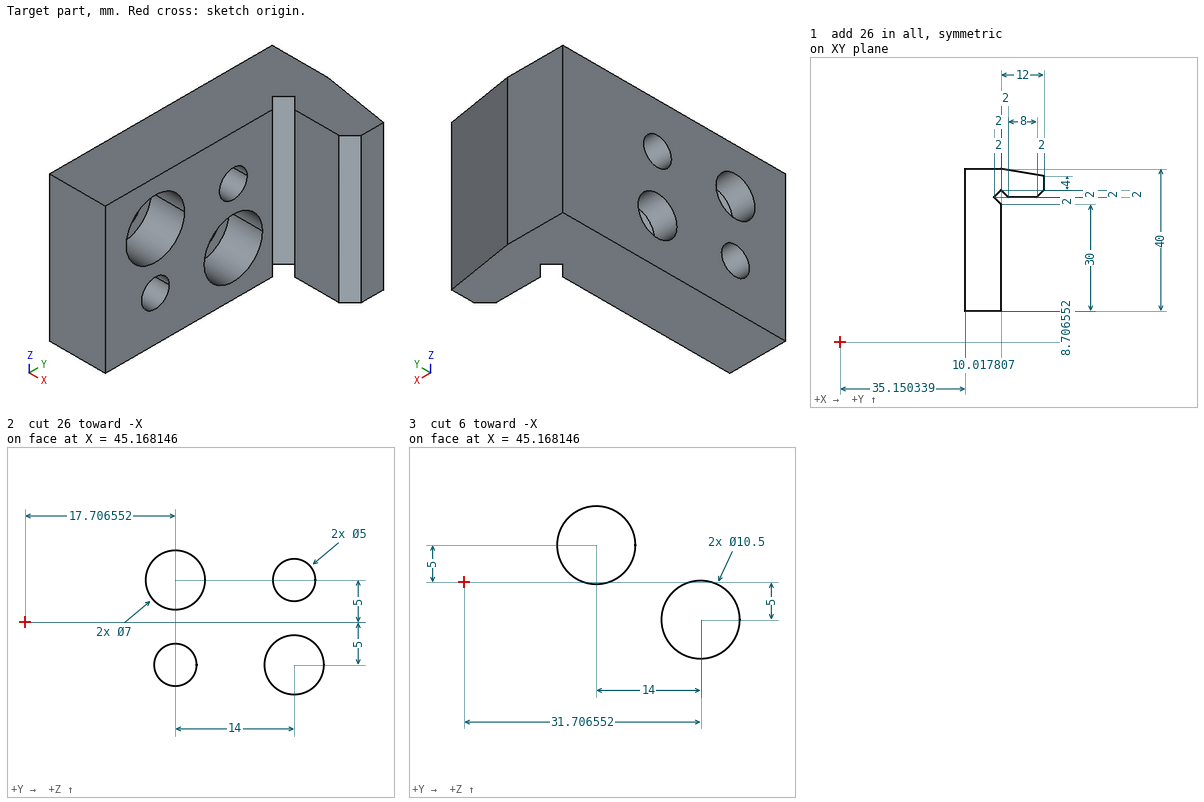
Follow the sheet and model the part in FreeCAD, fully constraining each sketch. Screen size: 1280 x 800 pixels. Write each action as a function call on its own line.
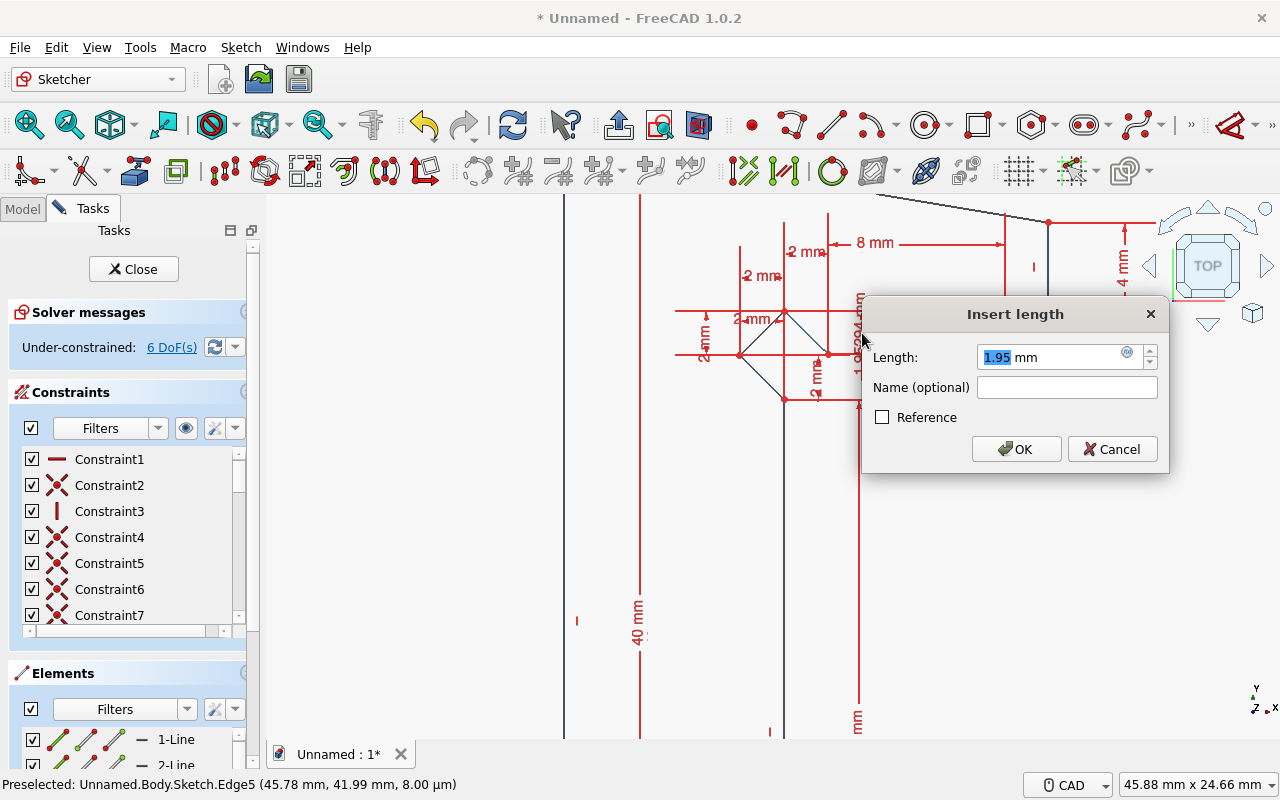
text(2)
key(Return)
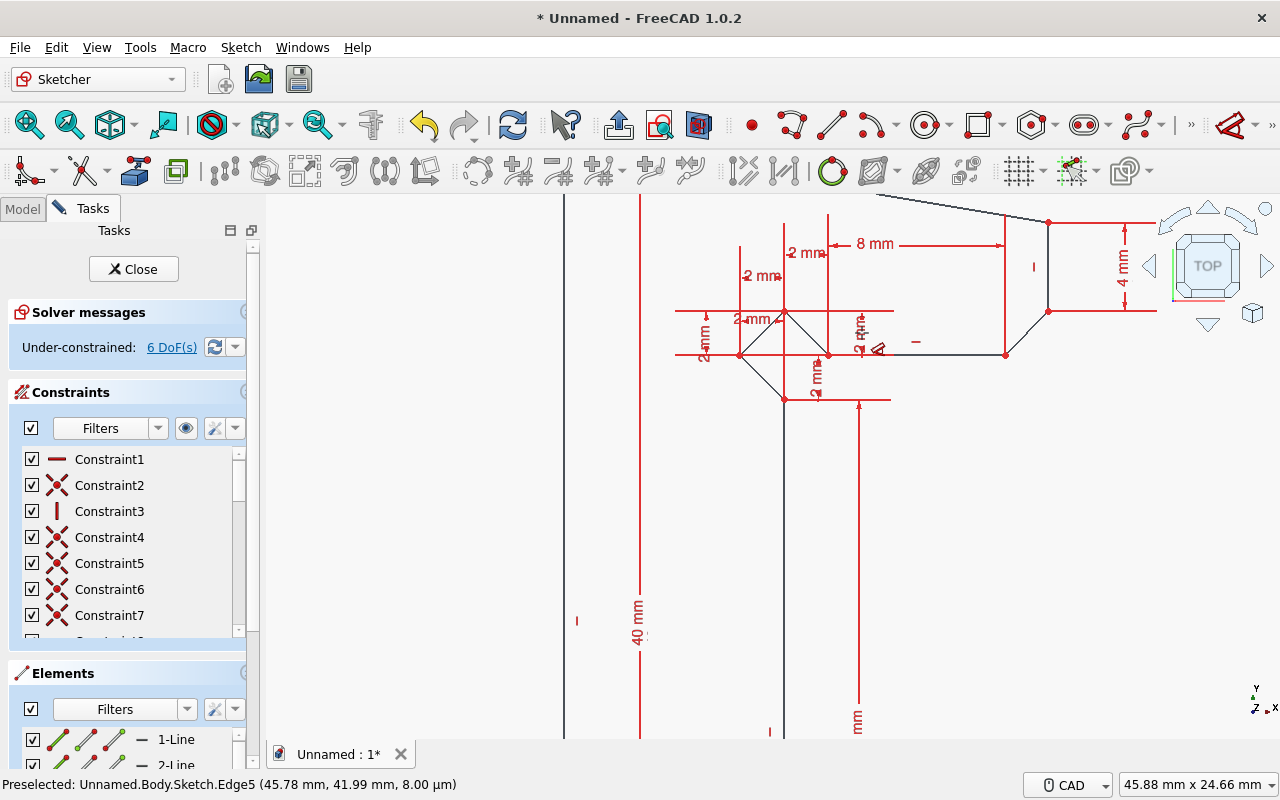
click(1018, 342)
click(1027, 277)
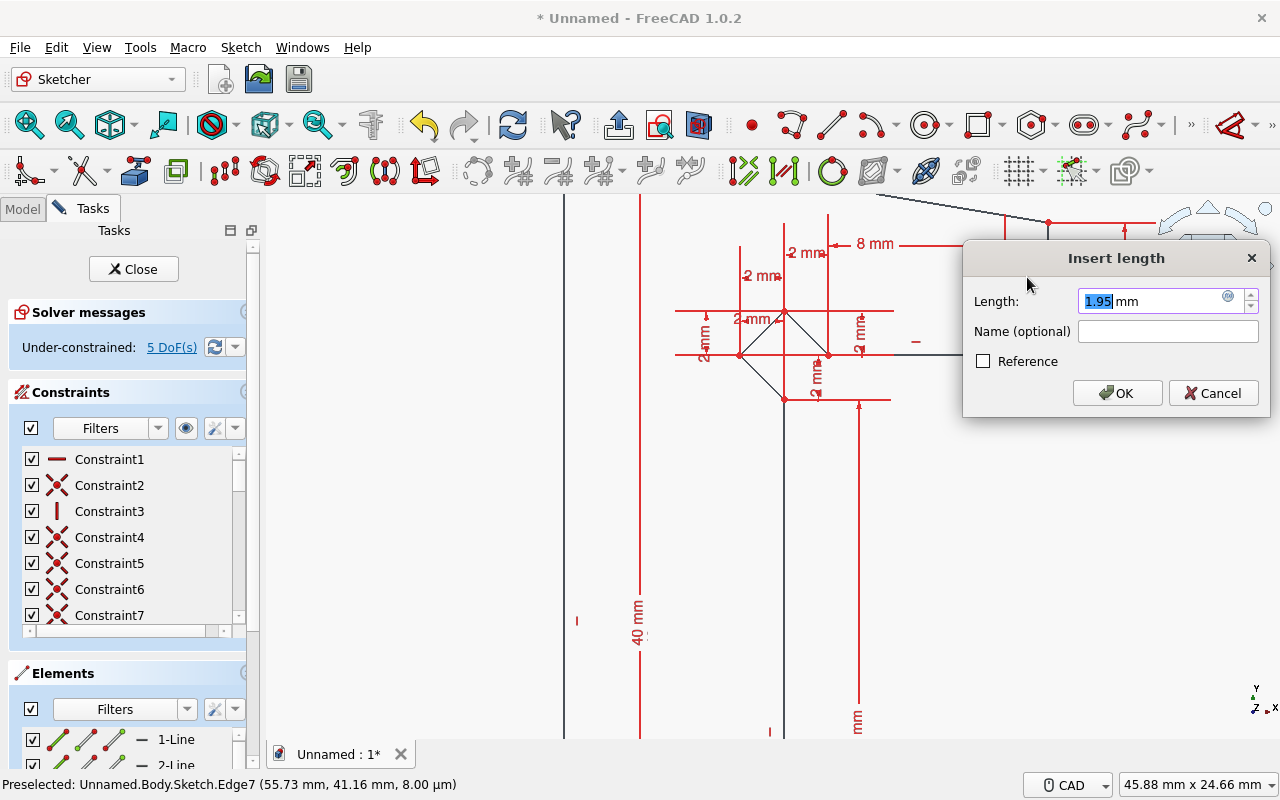
text(2)
key(Return)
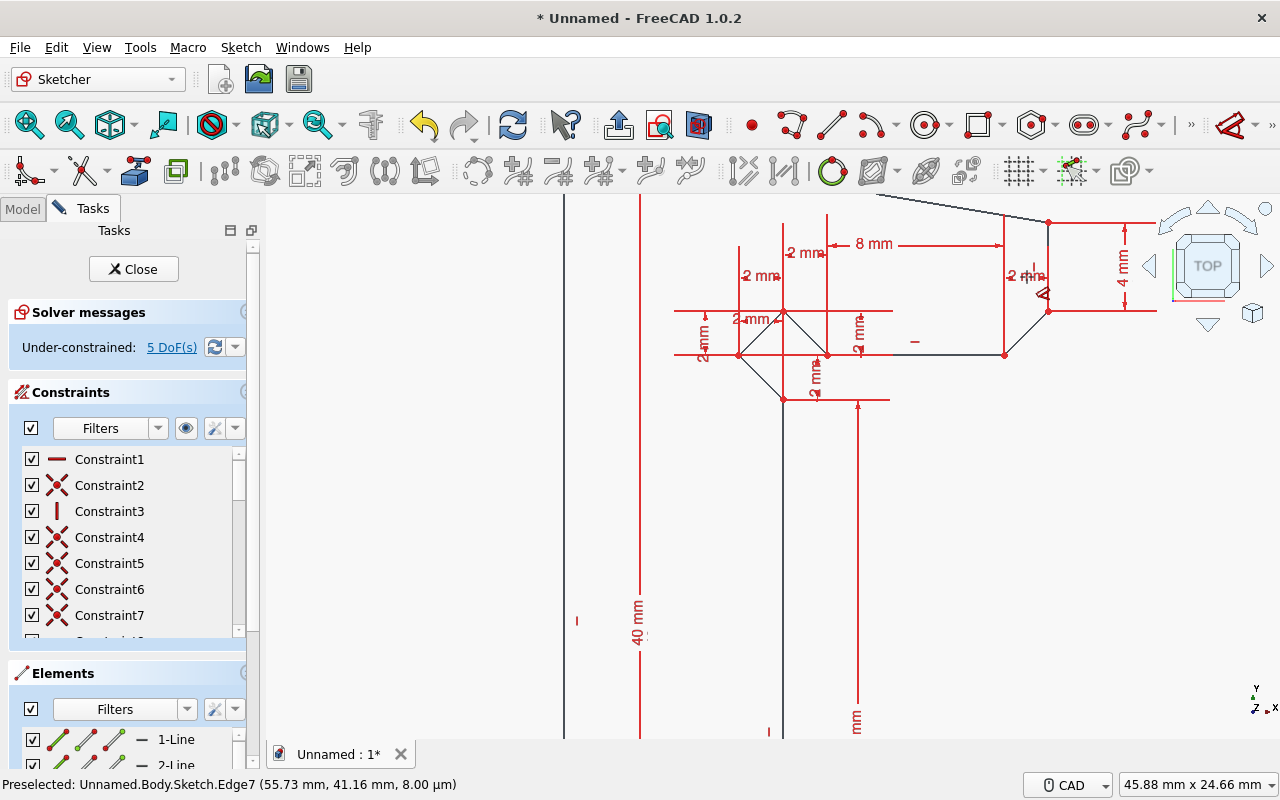
click(1017, 342)
click(1082, 333)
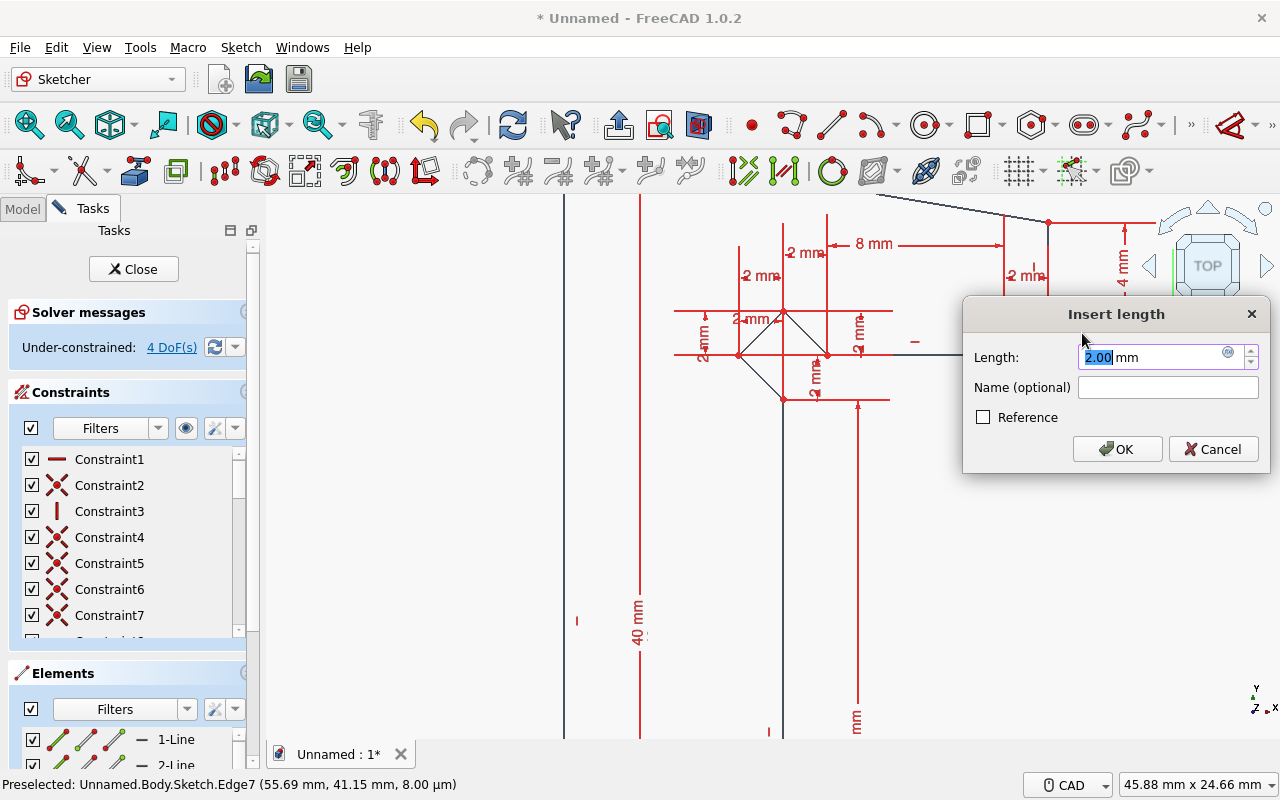
text(2)
key(Return)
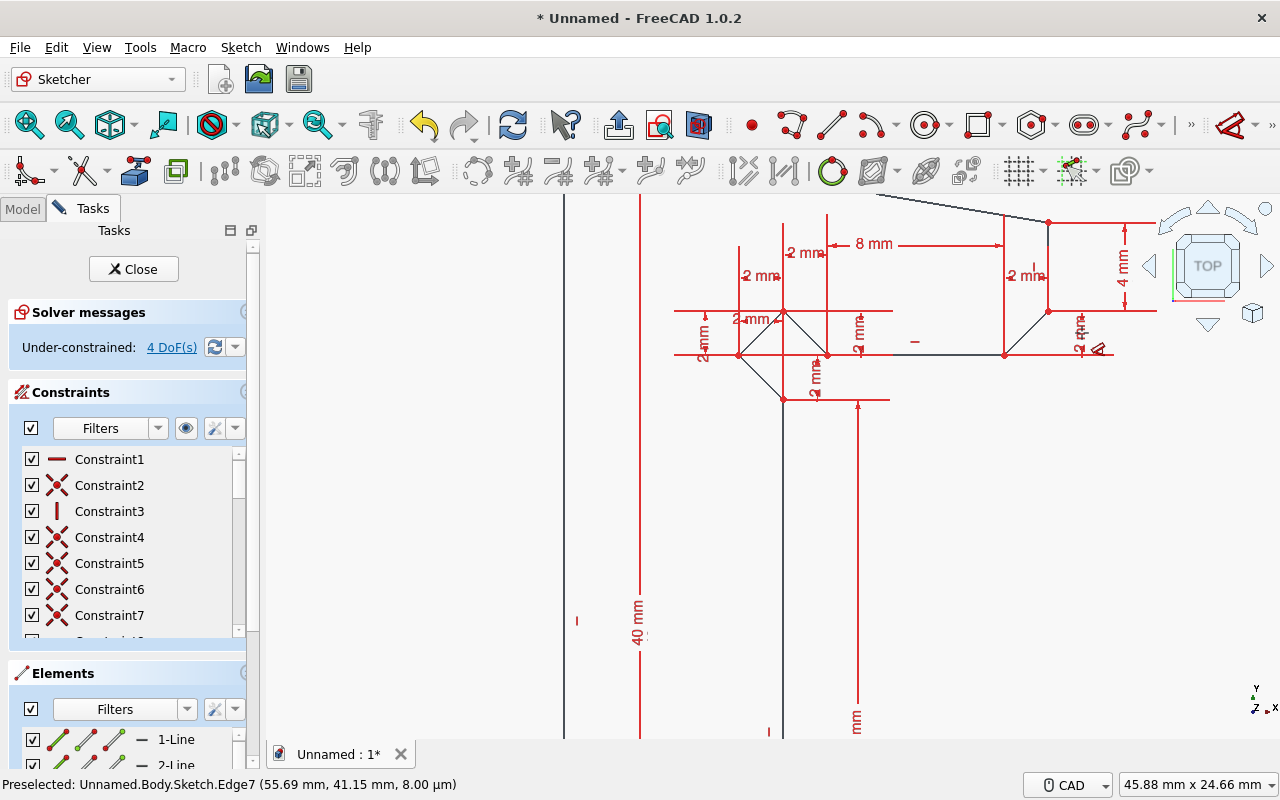
scroll(828, 360, down, 6)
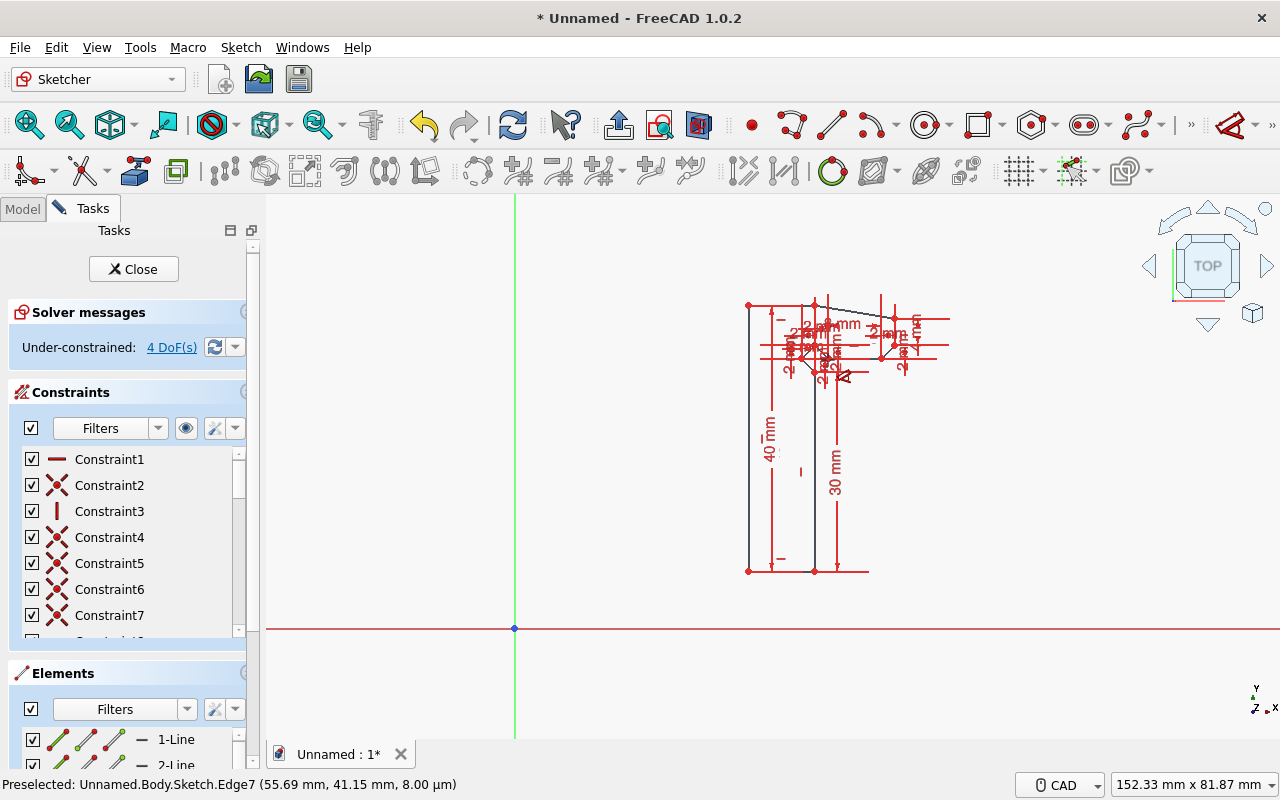
click(871, 315)
click(855, 272)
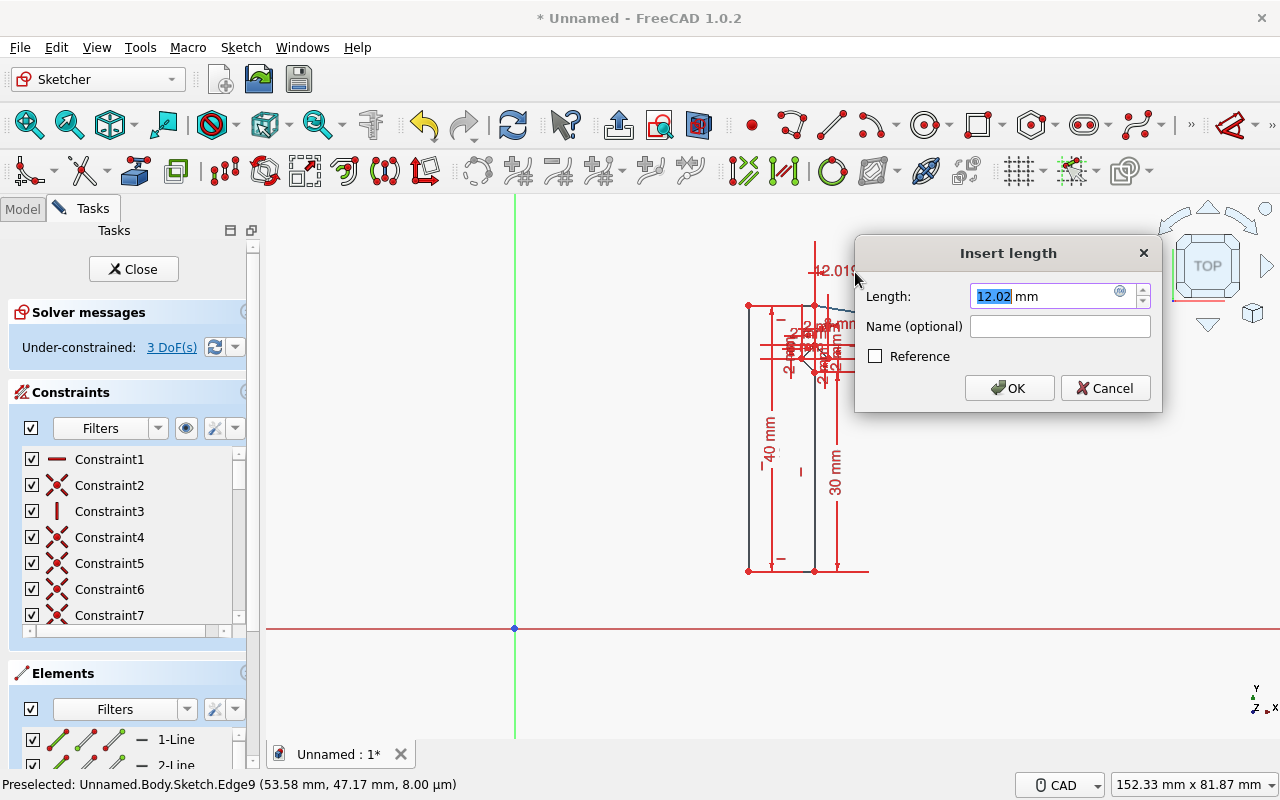
text(12)
key(Return)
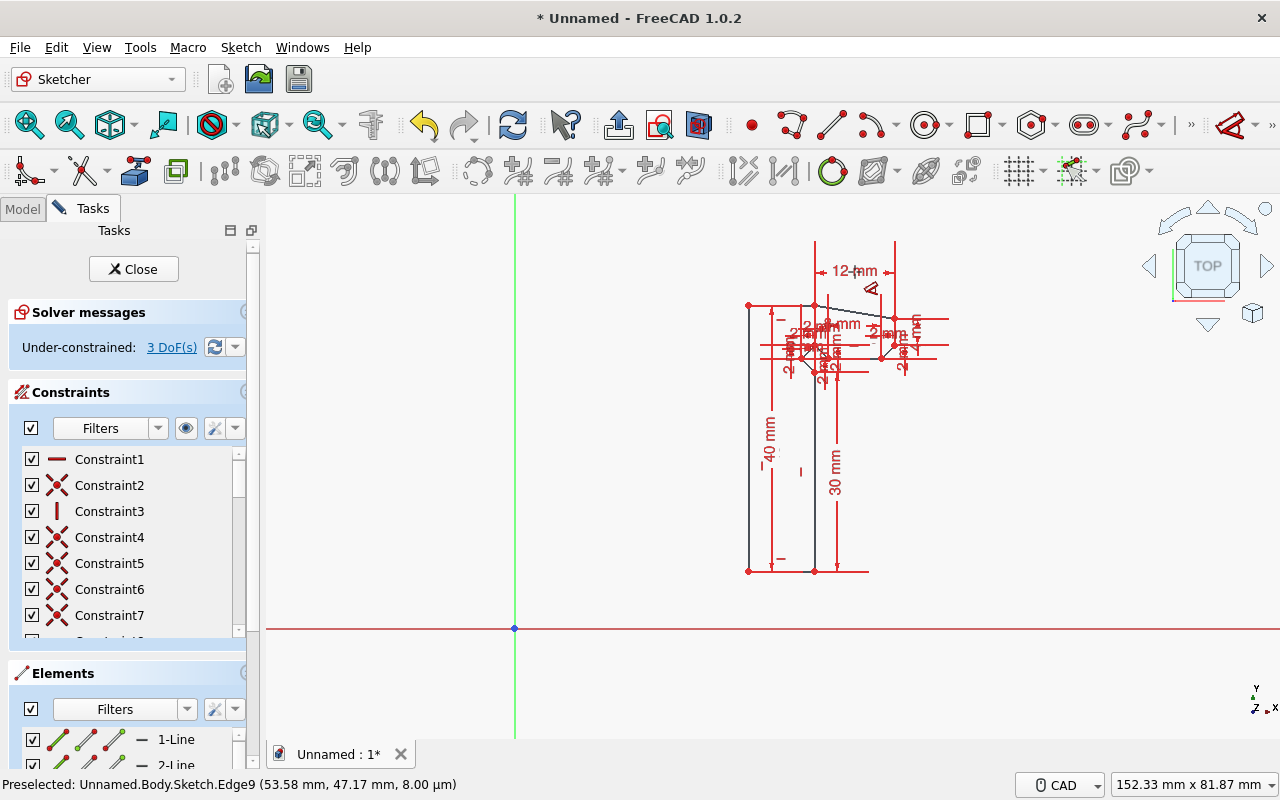
click(769, 572)
click(782, 606)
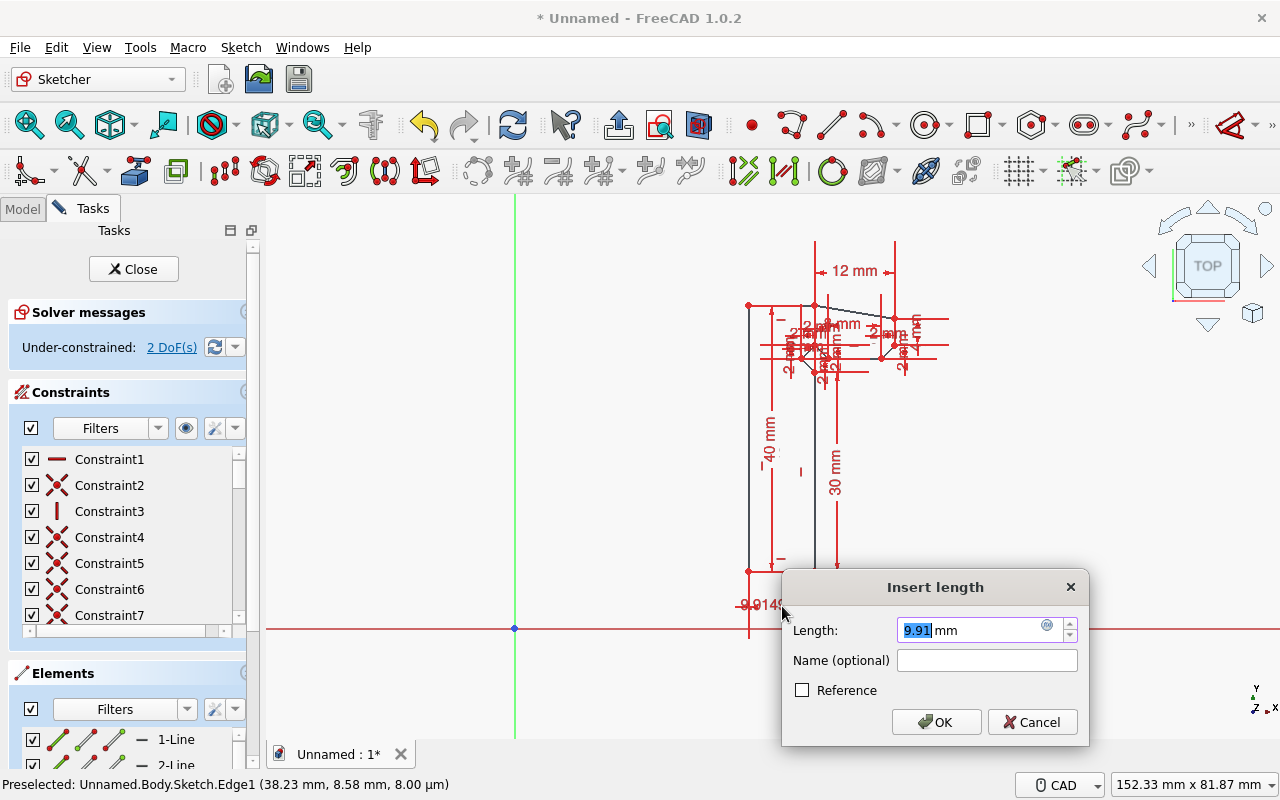
text(10.017807)
key(Return)